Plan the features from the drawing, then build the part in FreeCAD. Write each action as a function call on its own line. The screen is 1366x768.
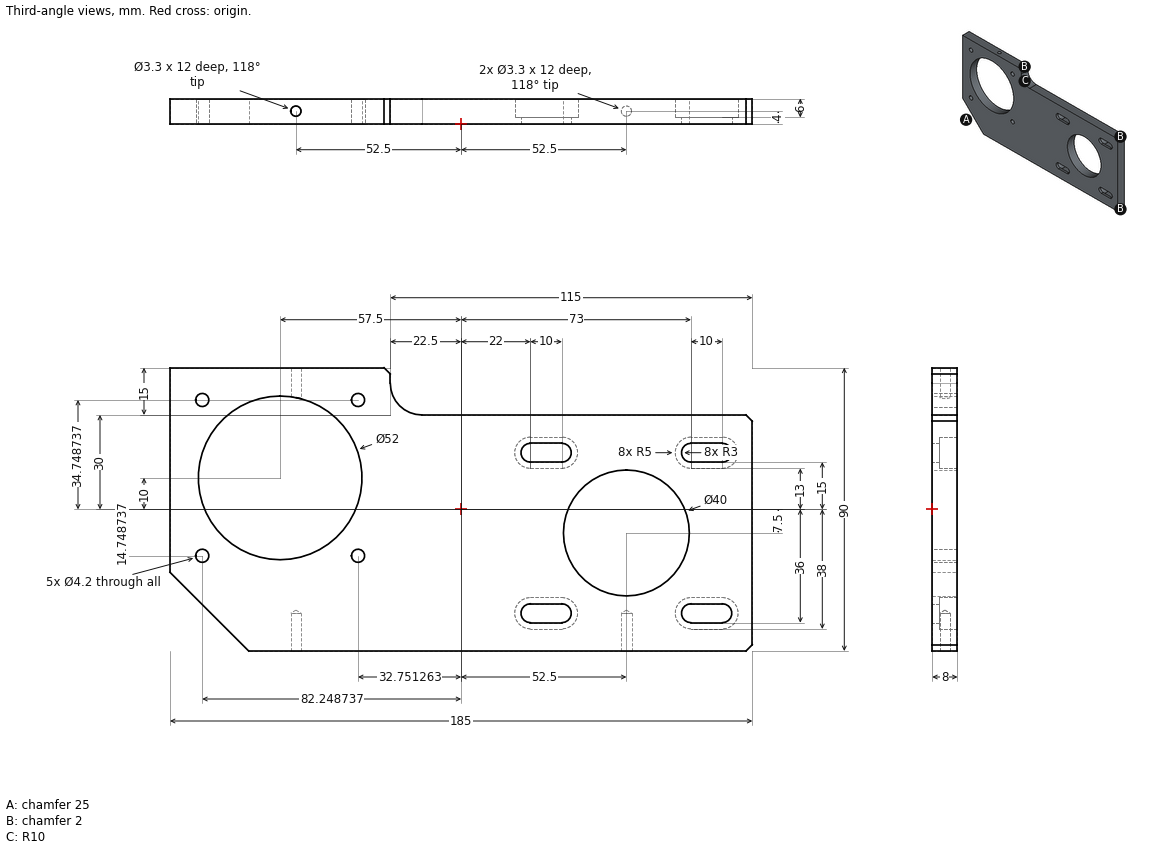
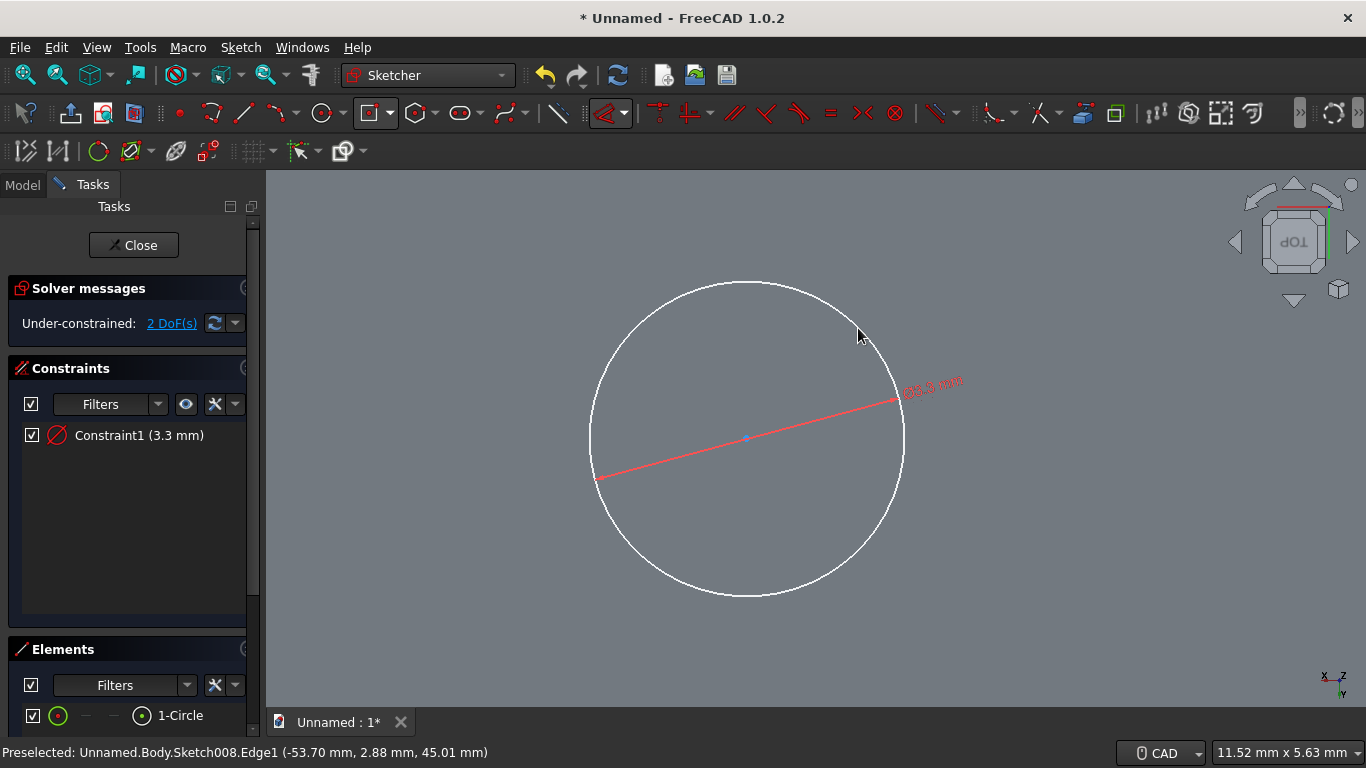
click(747, 439)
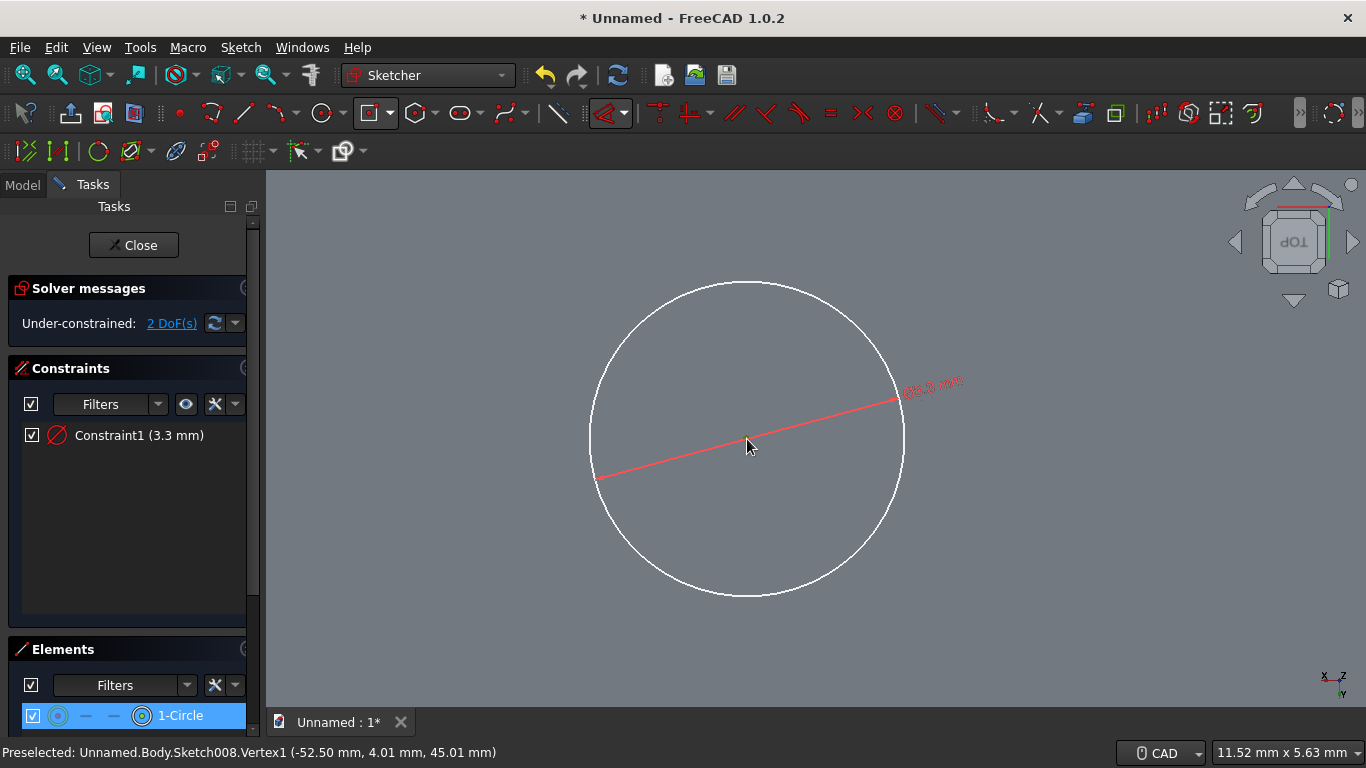
key(i)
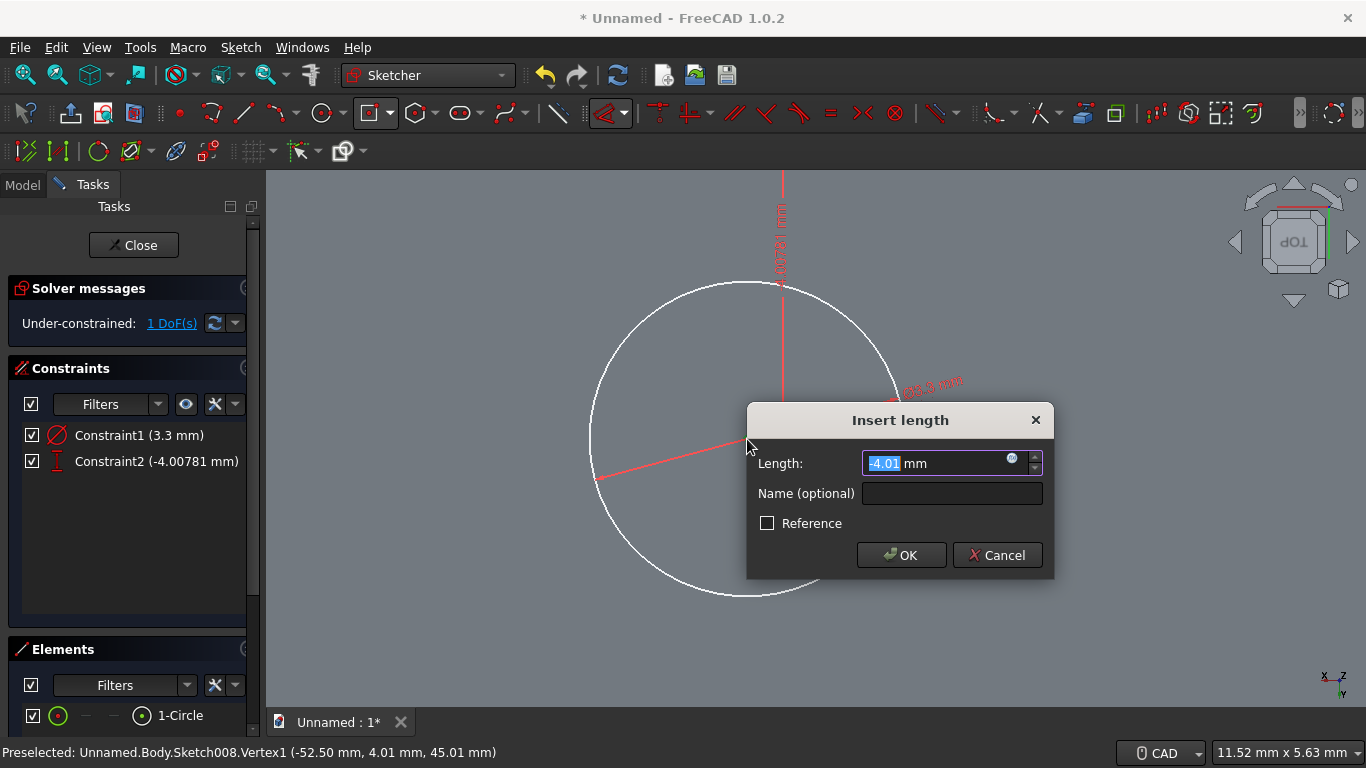
text(-4)
key(Return)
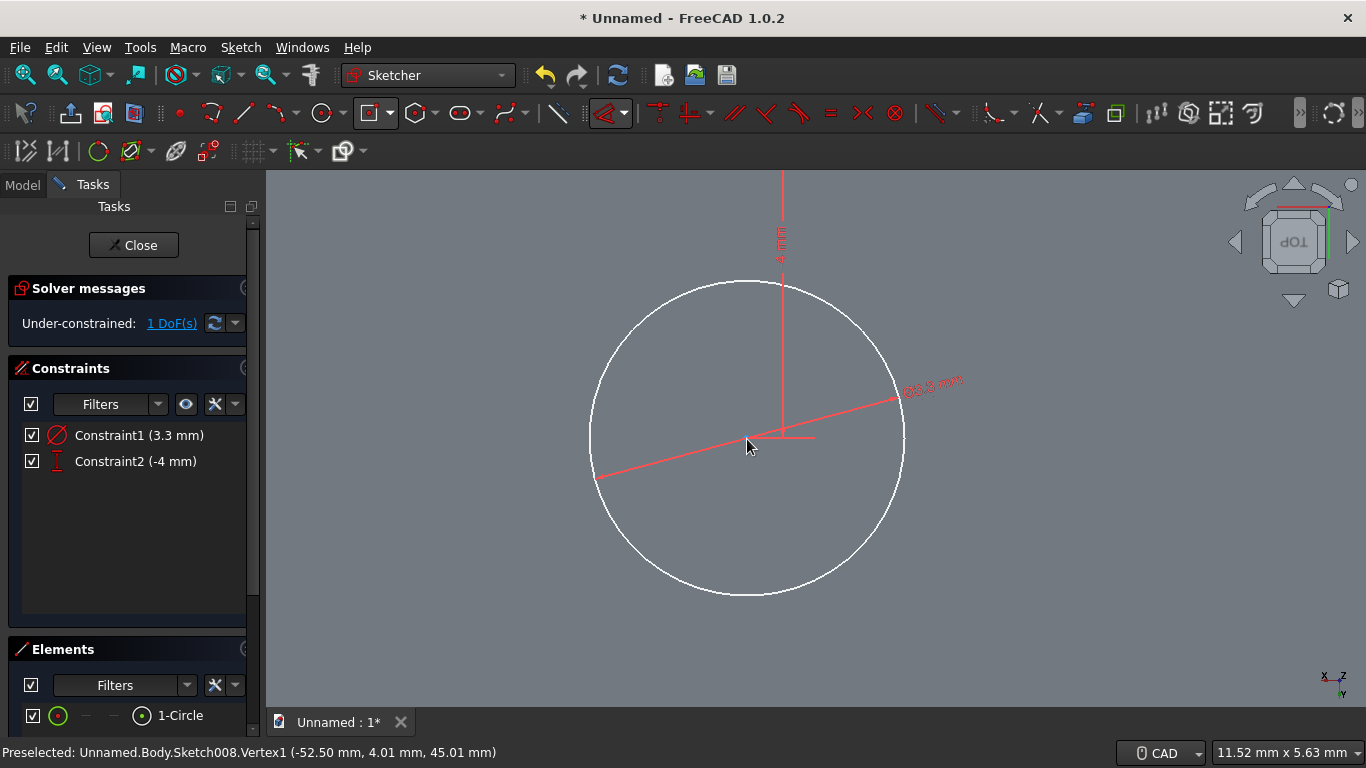
click(747, 438)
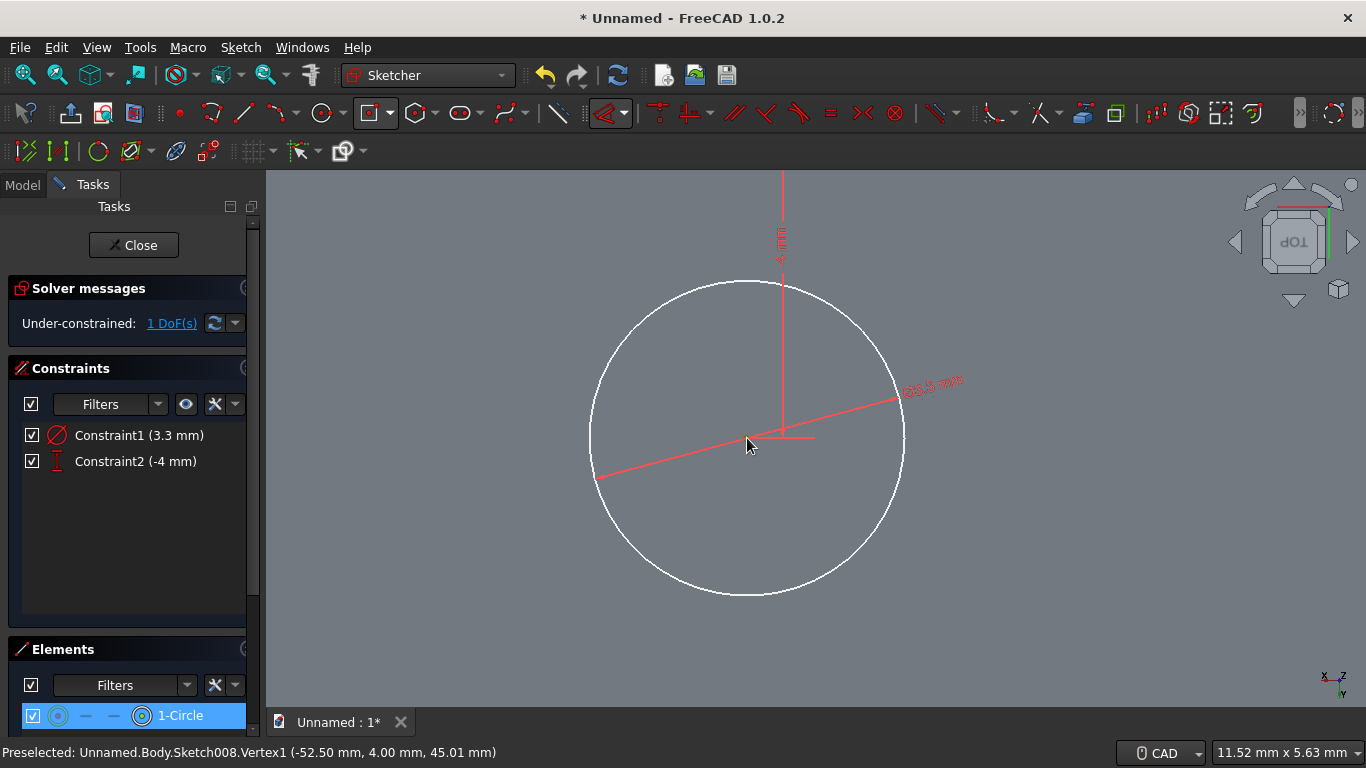
key(l)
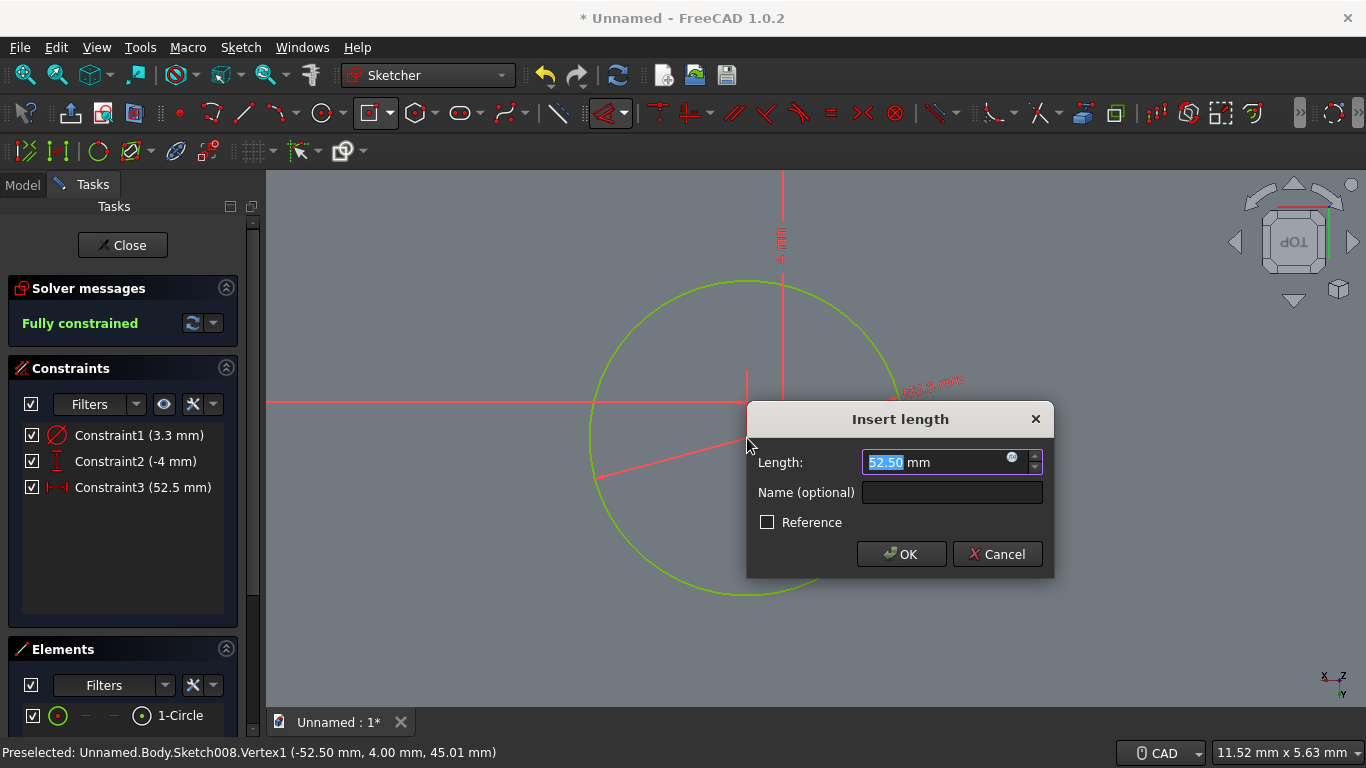
text(52.5)
key(Return)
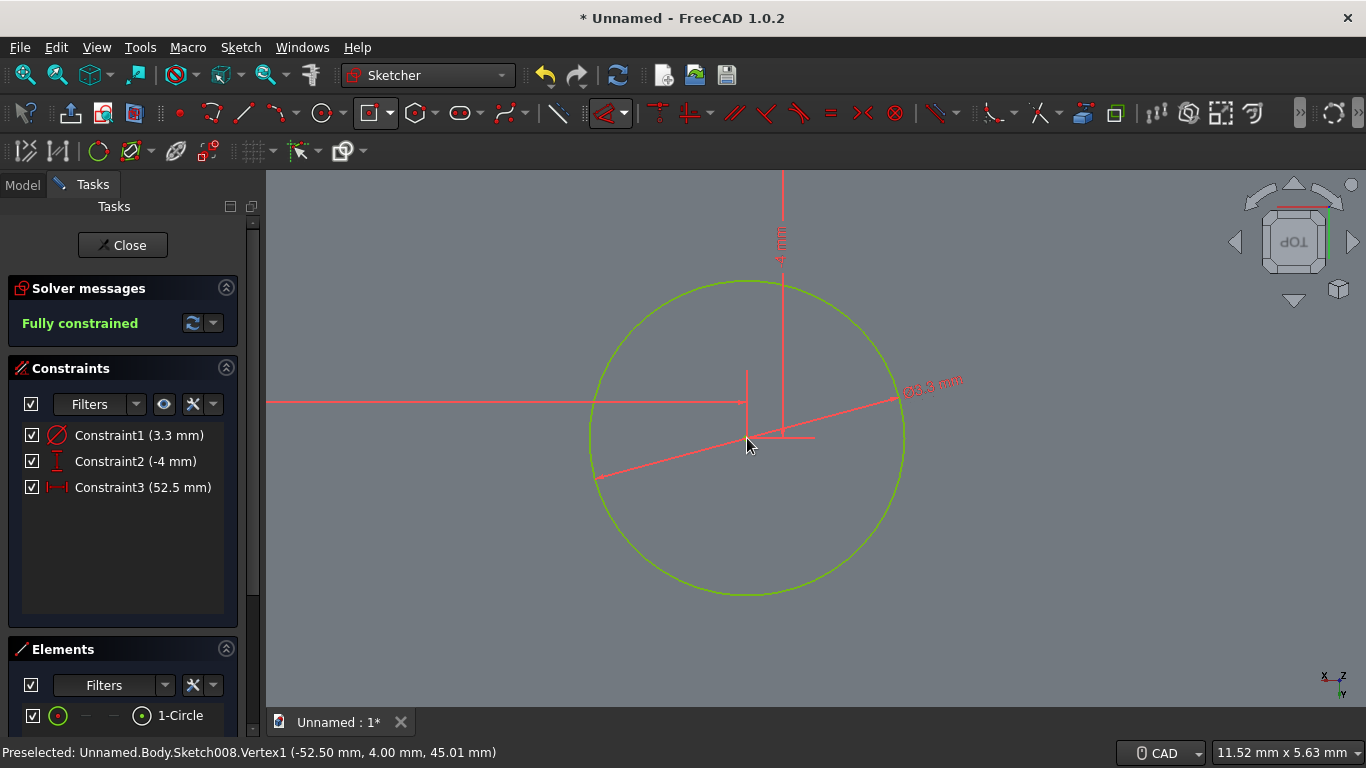
click(123, 245)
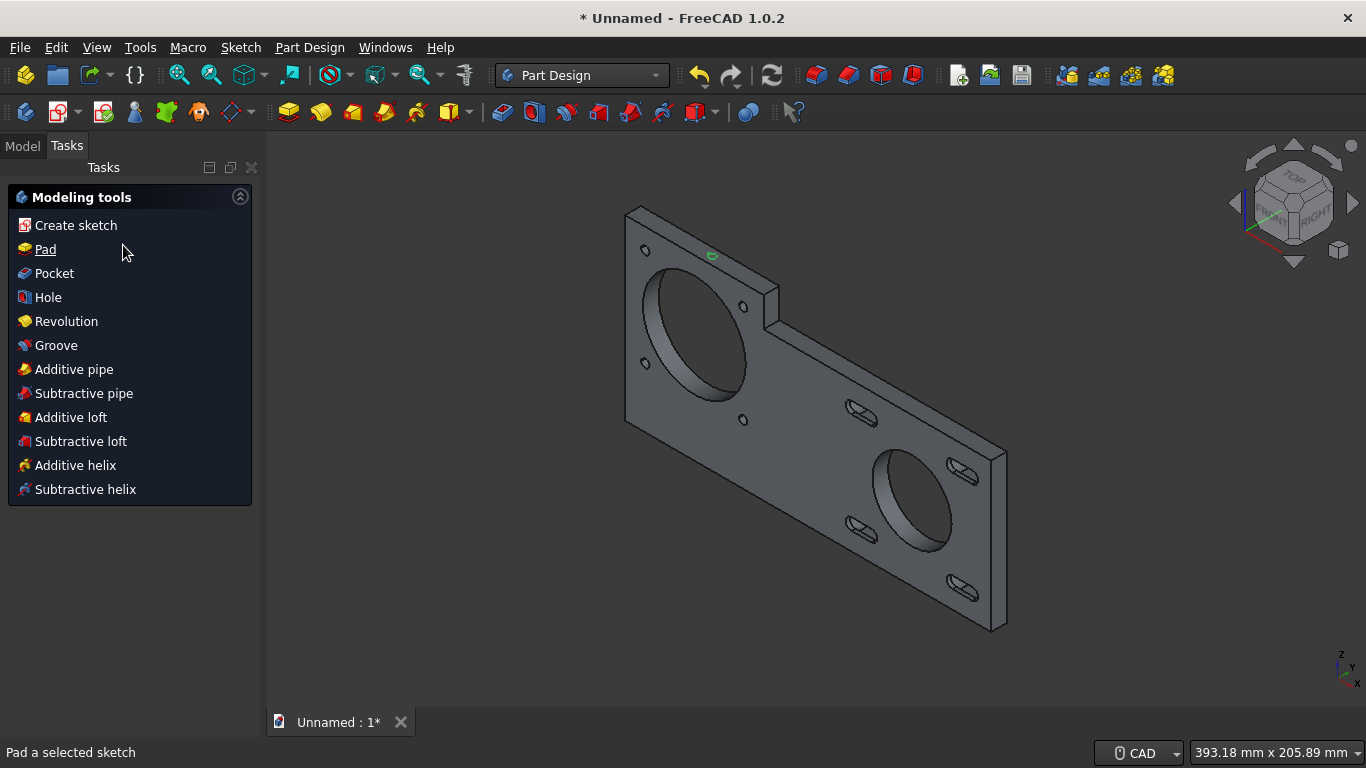
click(536, 112)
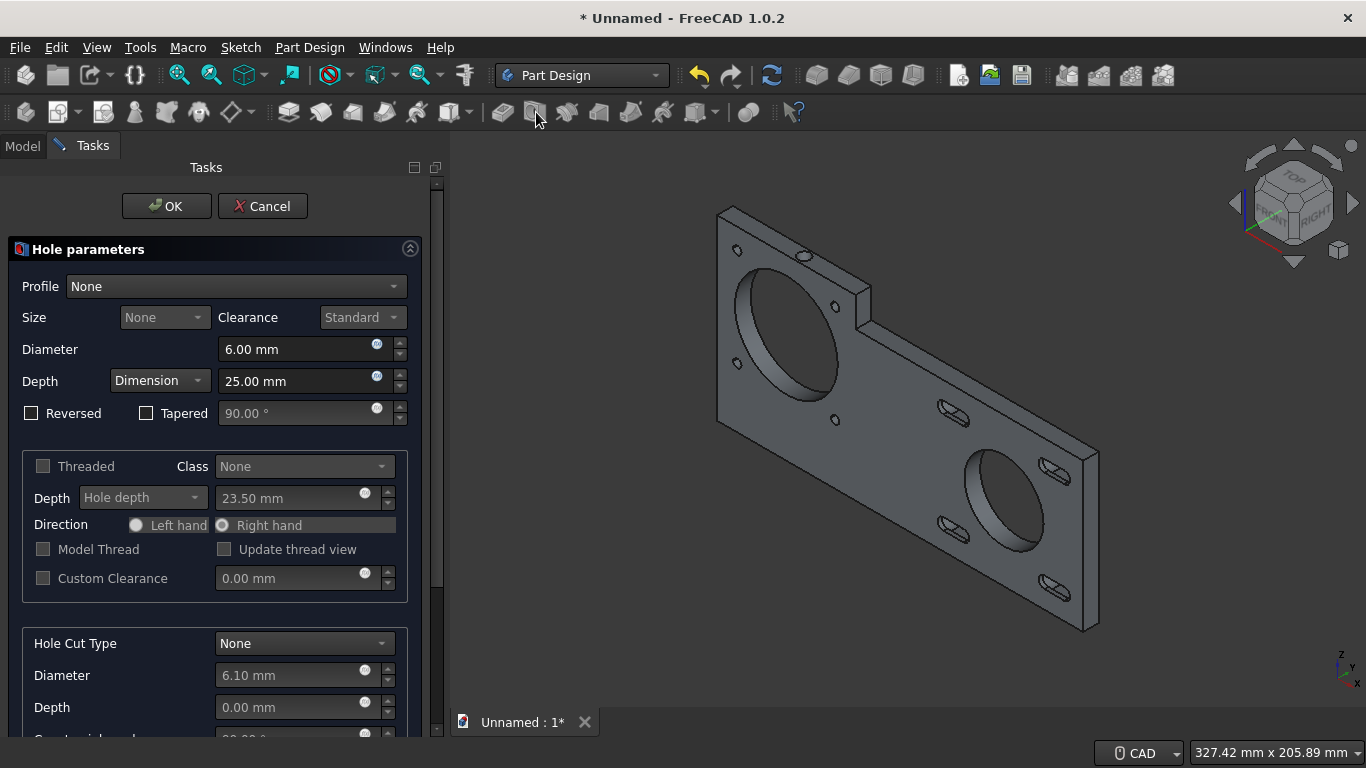
triple_click(305, 349)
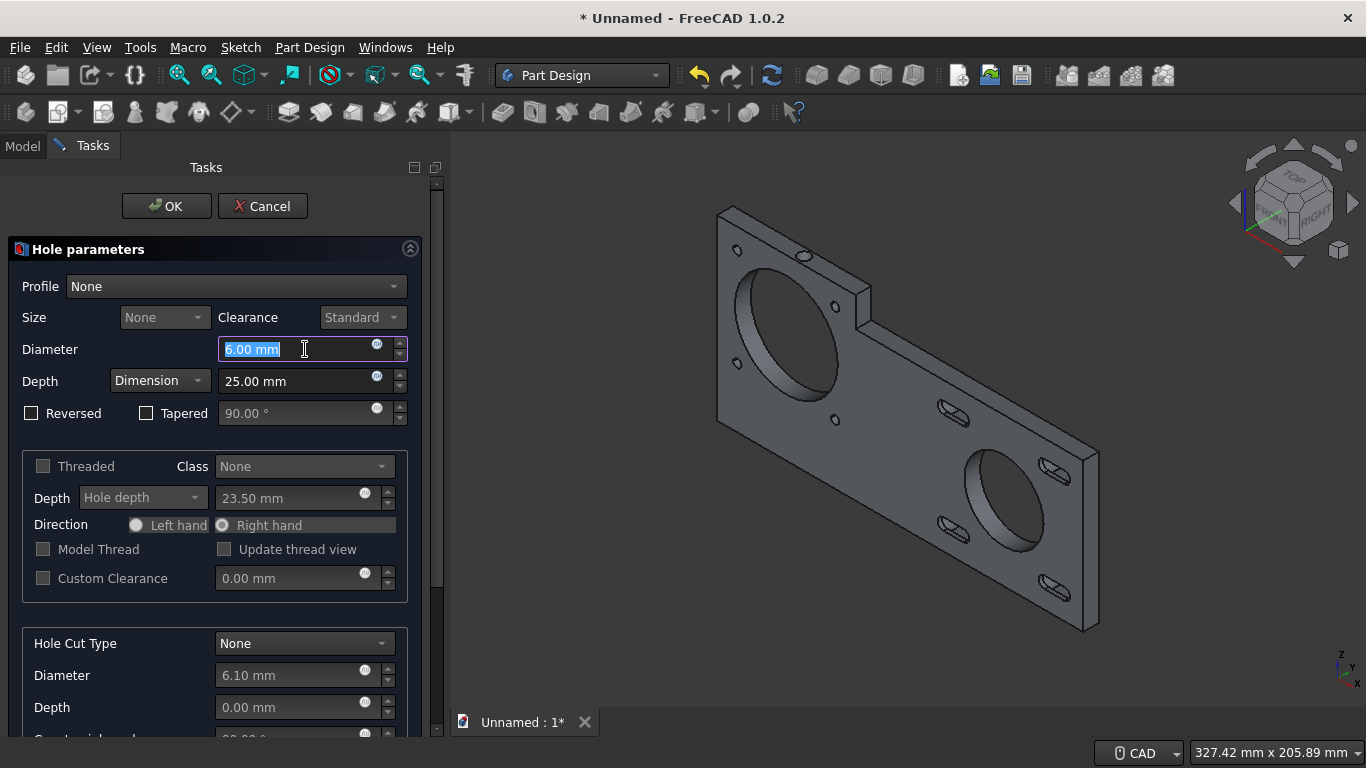
text(3.3)
key(Tab)